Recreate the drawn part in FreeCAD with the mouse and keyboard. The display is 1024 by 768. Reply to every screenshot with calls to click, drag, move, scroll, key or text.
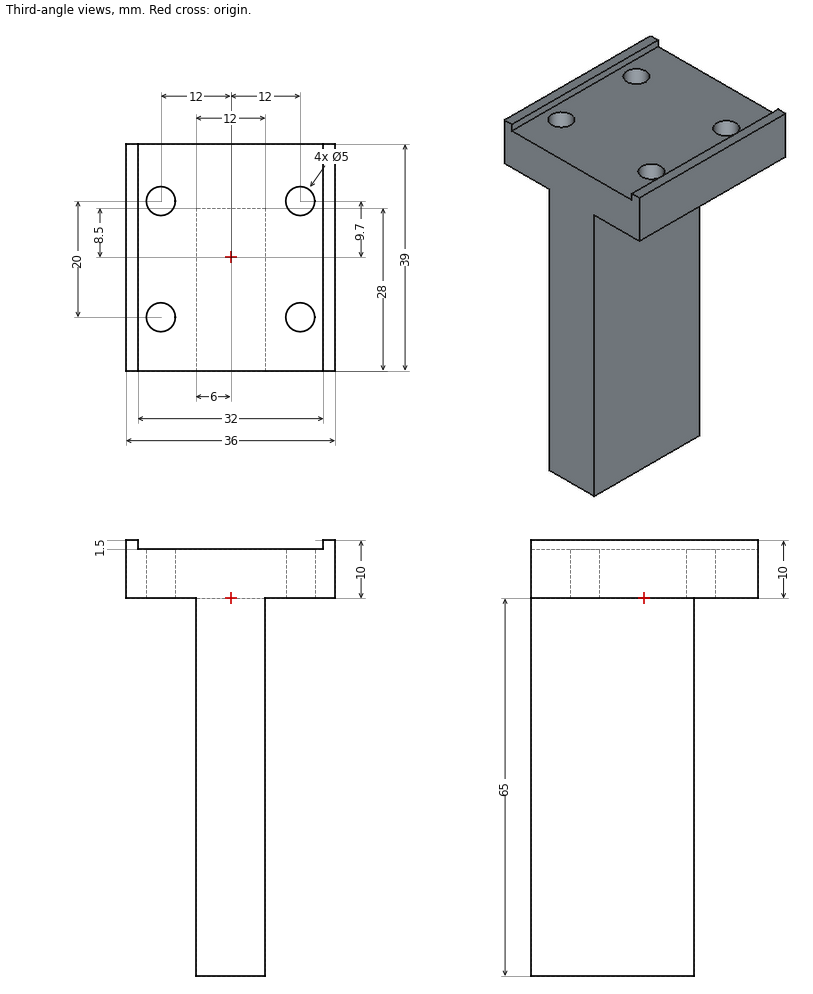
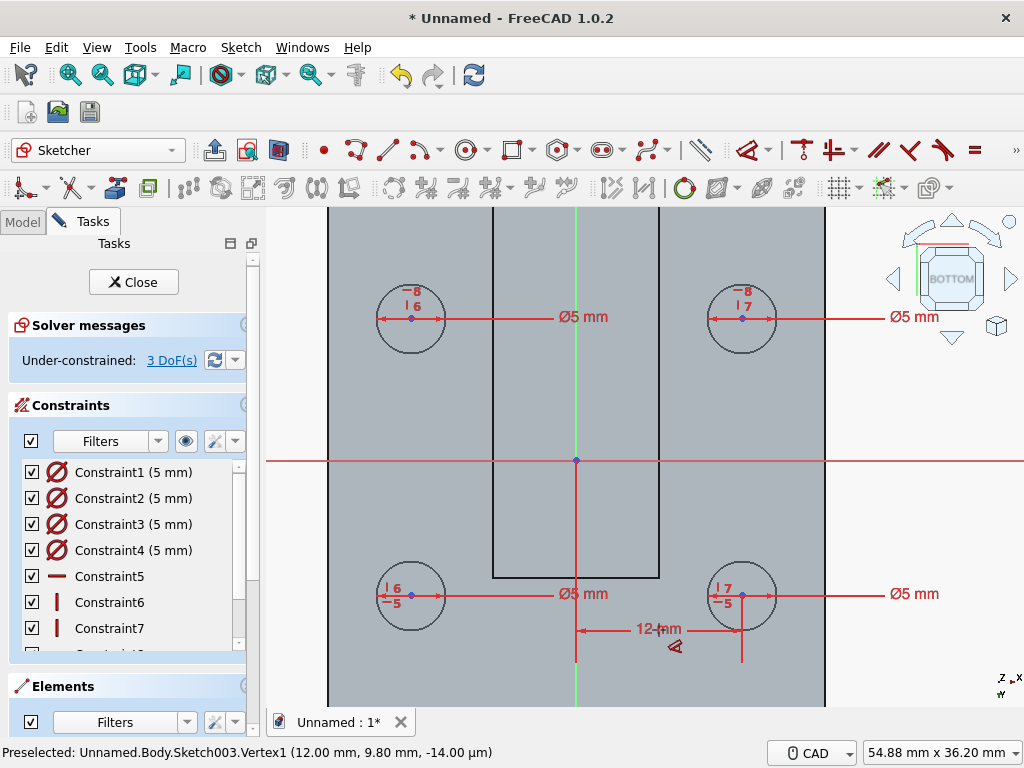
click(411, 596)
click(494, 630)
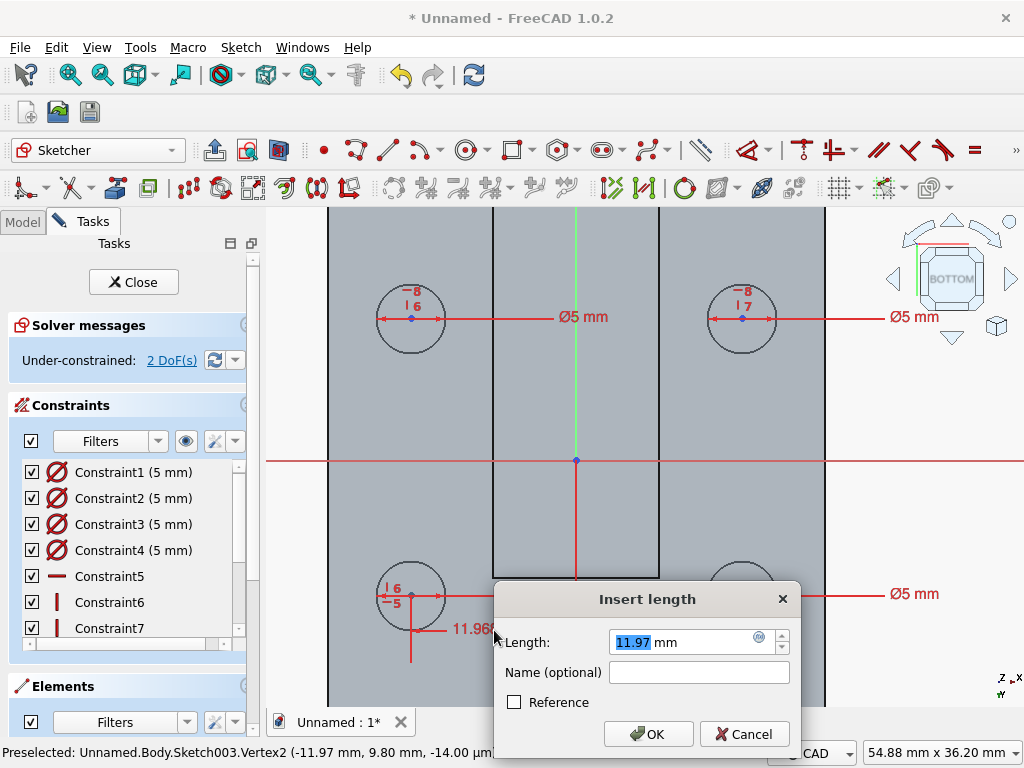
text(12)
key(Return)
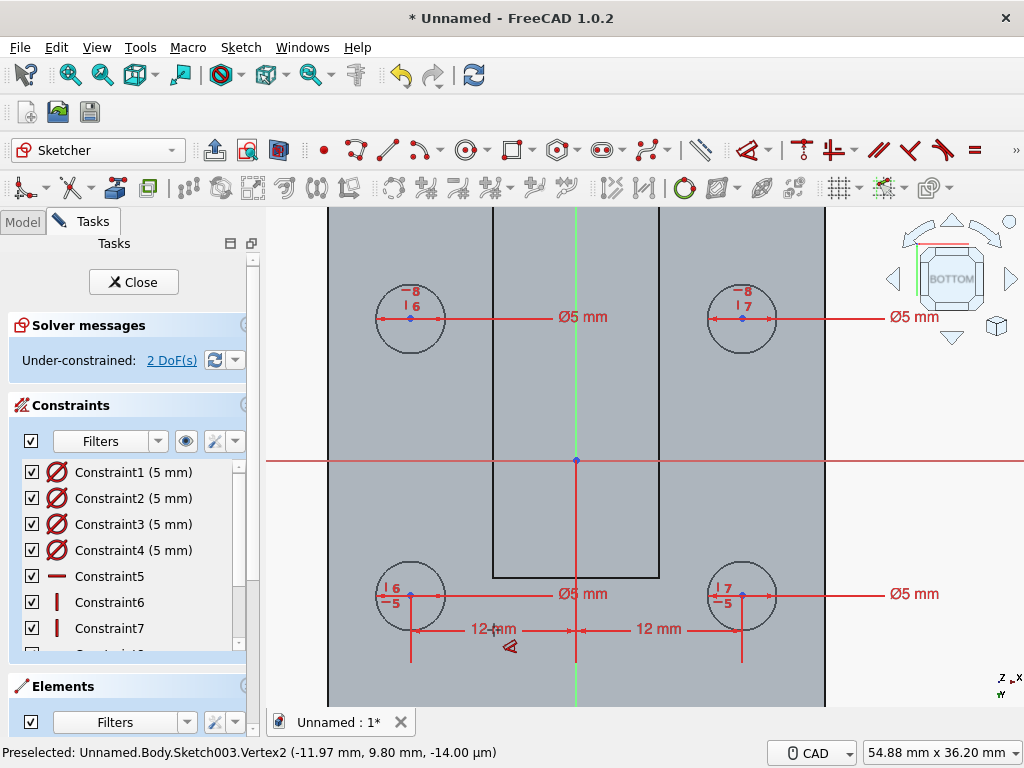
click(742, 596)
click(776, 528)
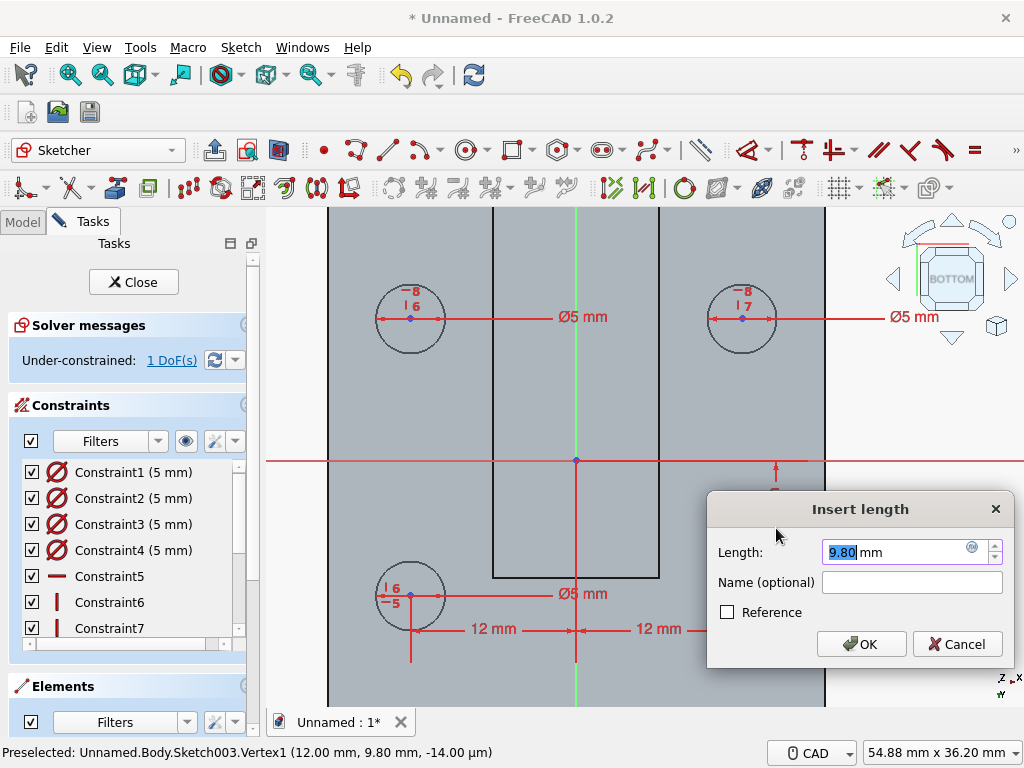
text(9.7)
key(Return)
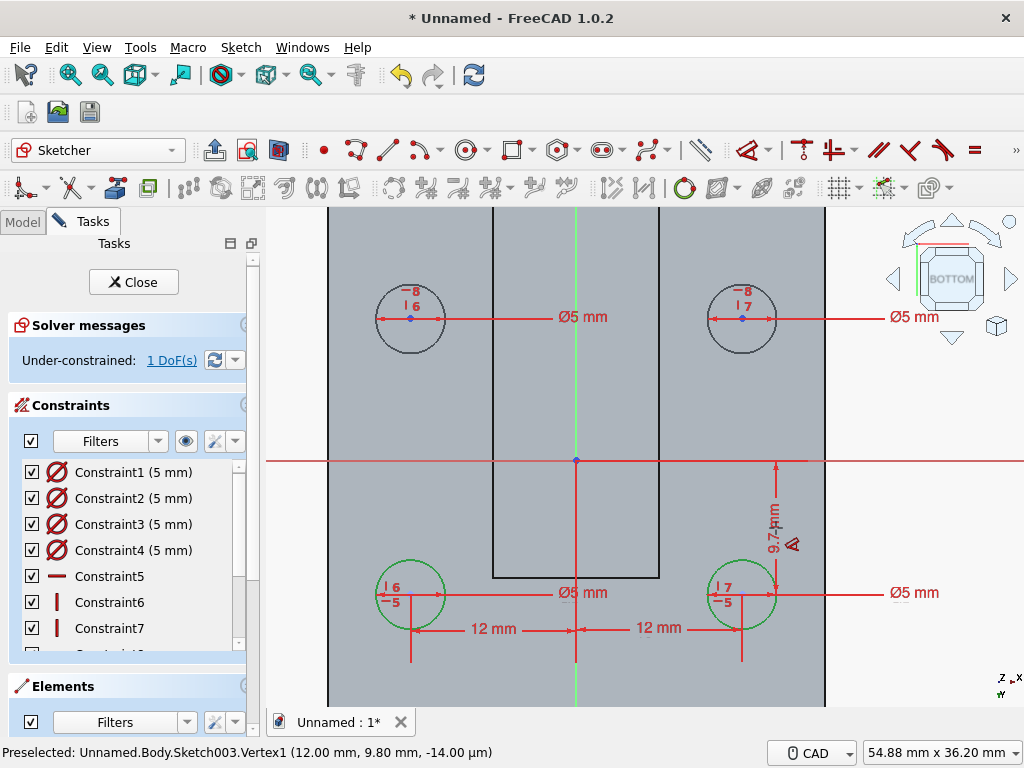
click(411, 595)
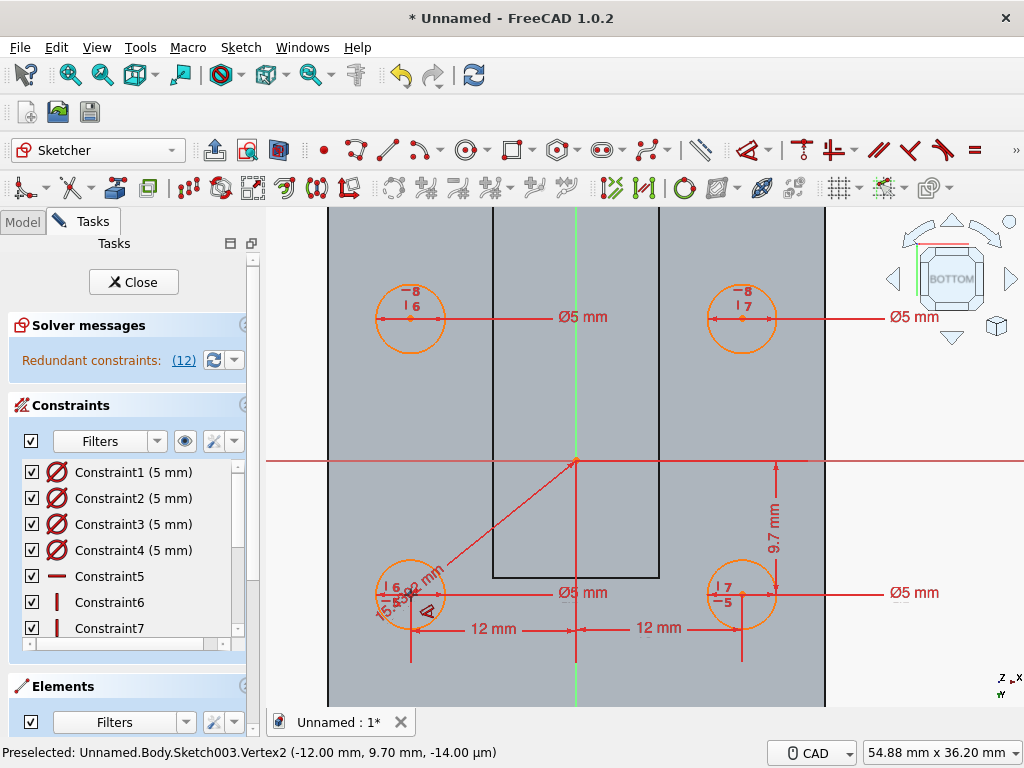
click(411, 319)
click(377, 393)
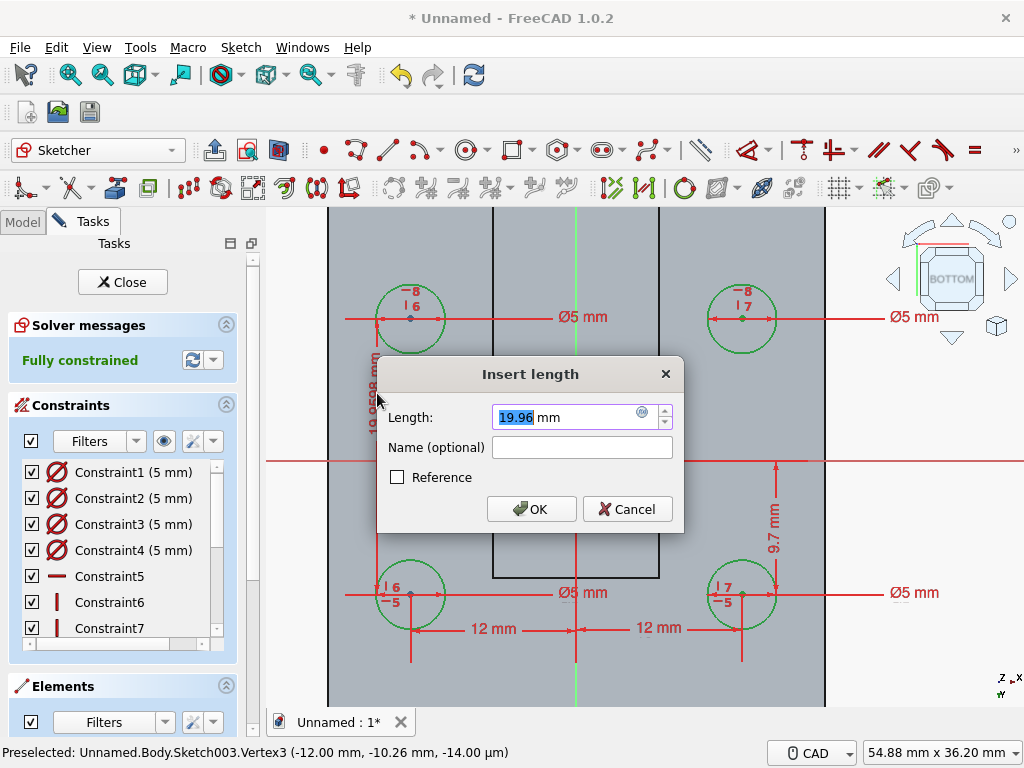
text(20)
key(Return)
key(Escape)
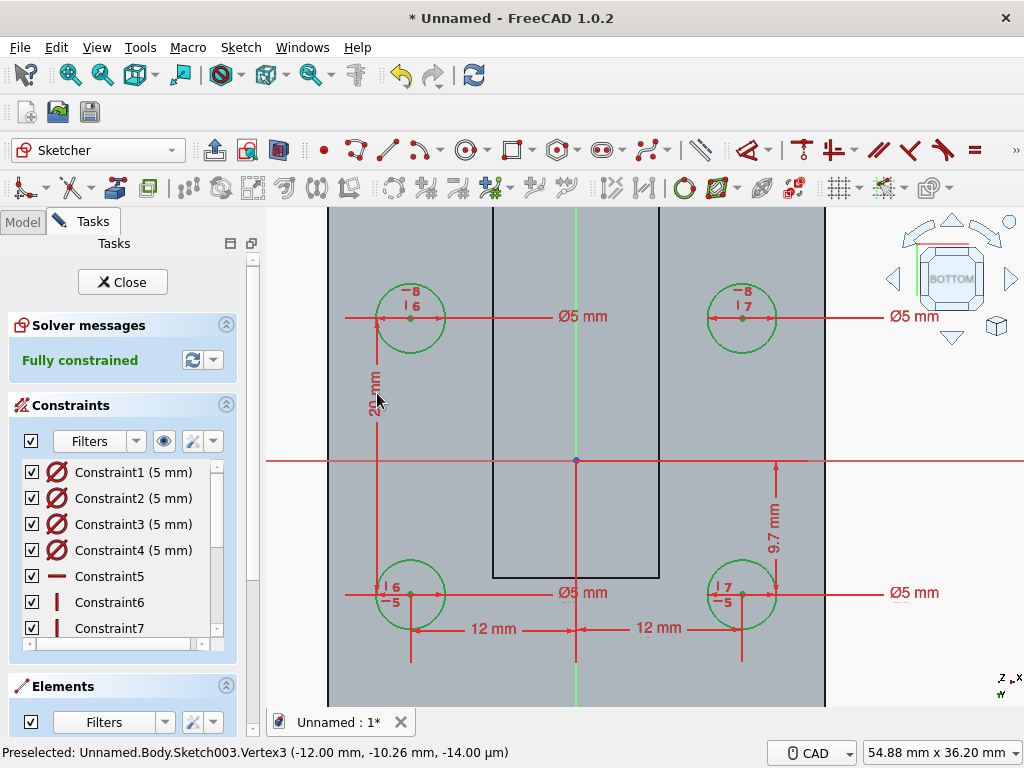
click(123, 282)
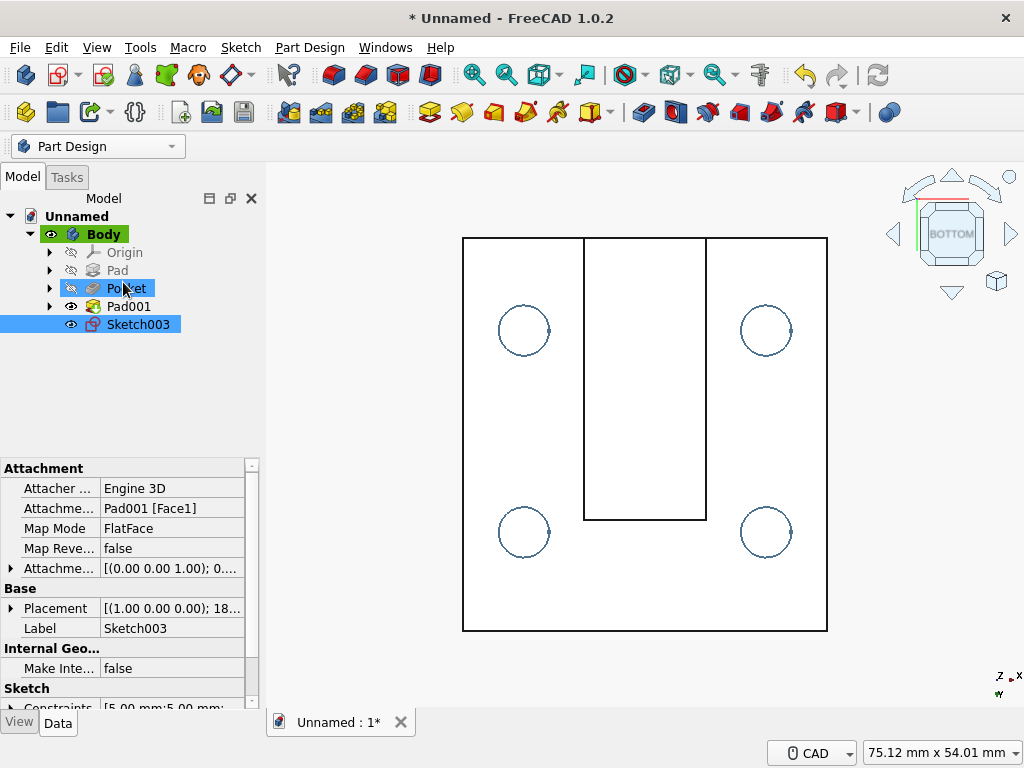
click(644, 112)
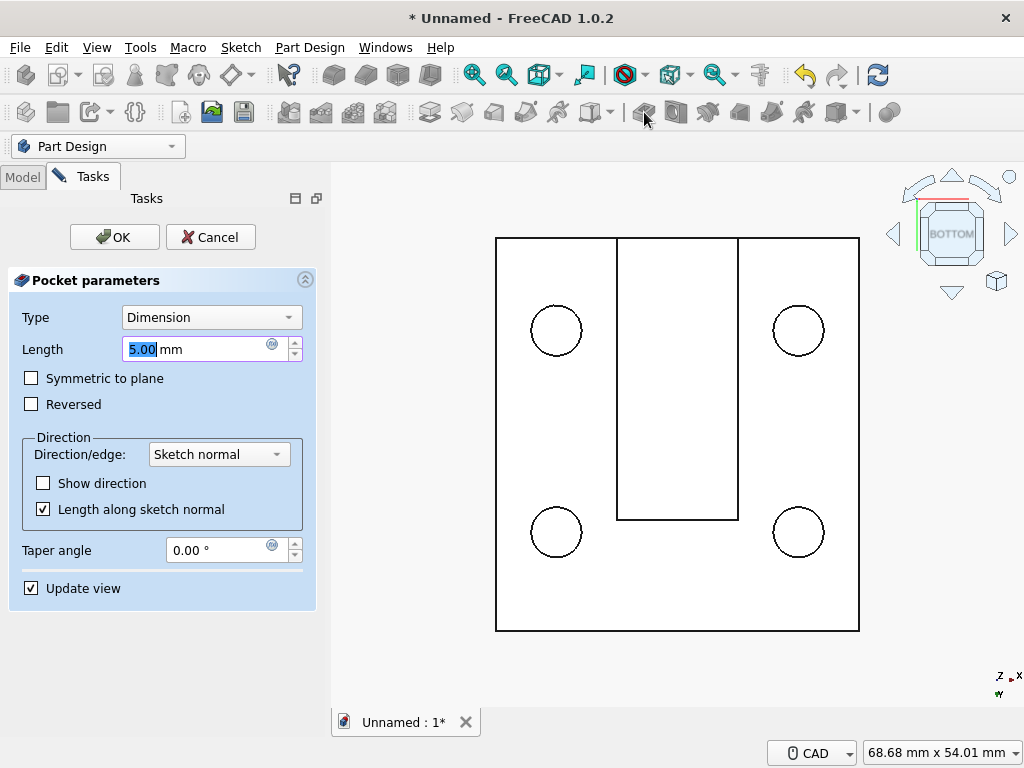
text(10)
key(Tab)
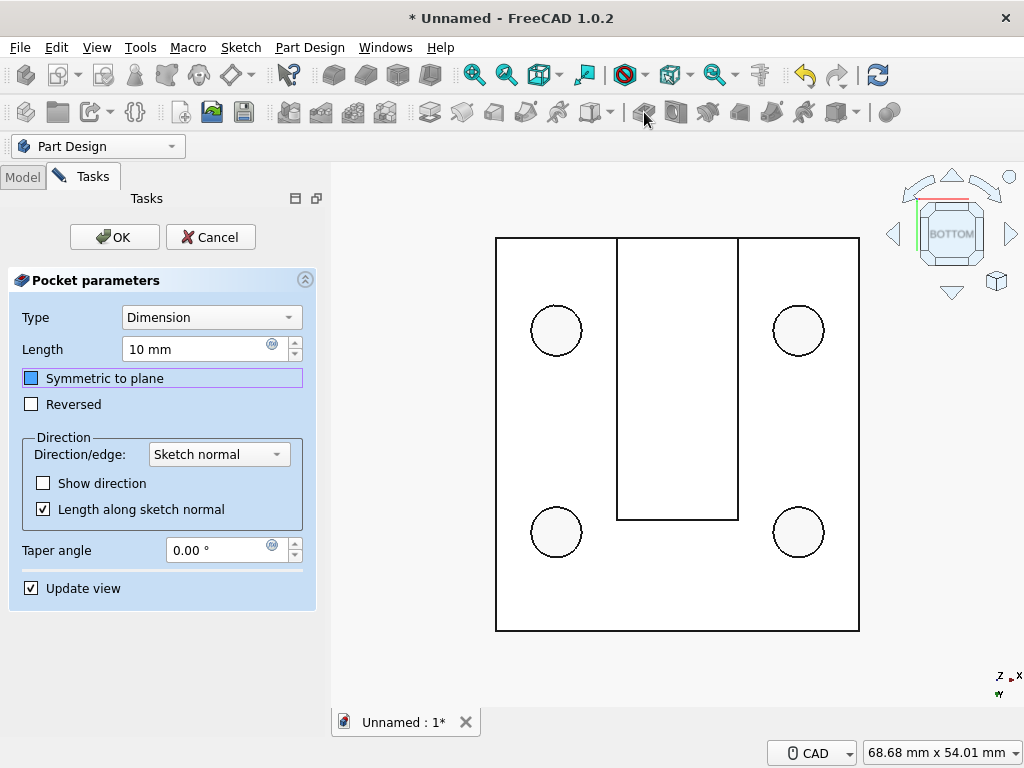
click(115, 237)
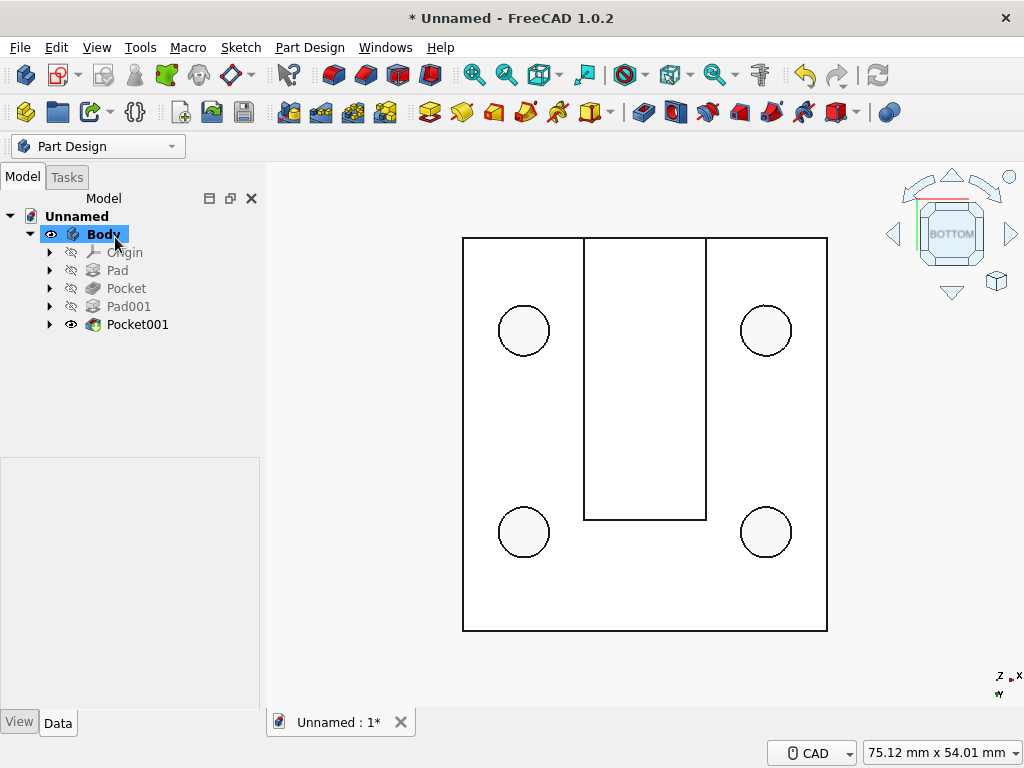
key(0)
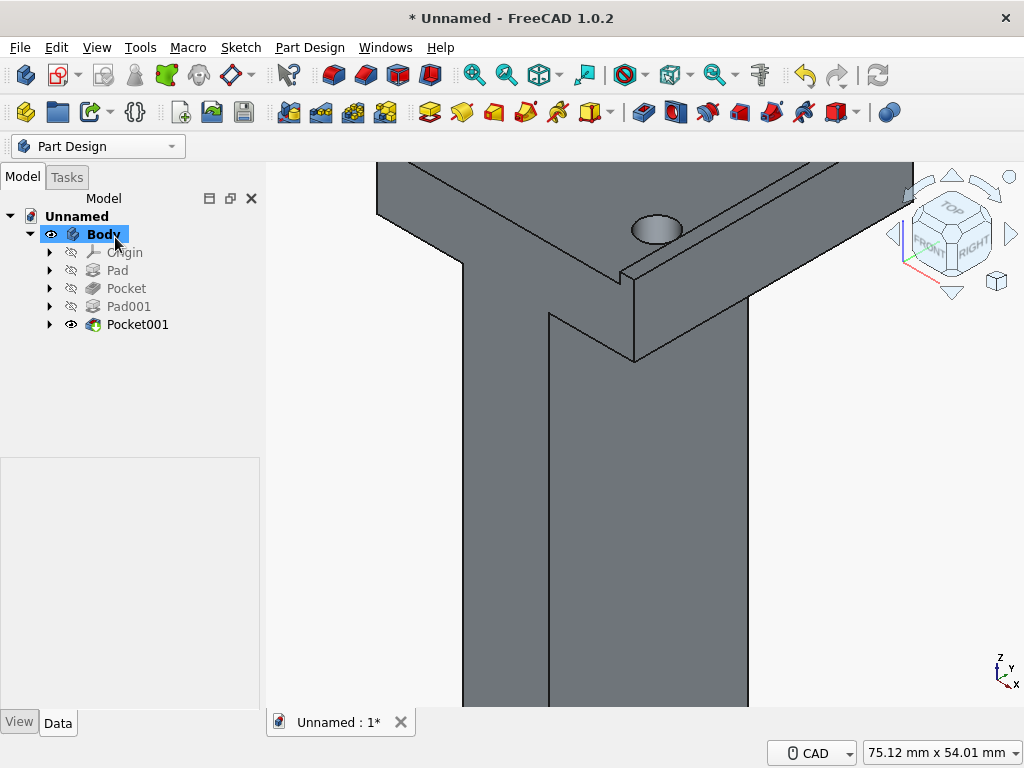
click(476, 76)